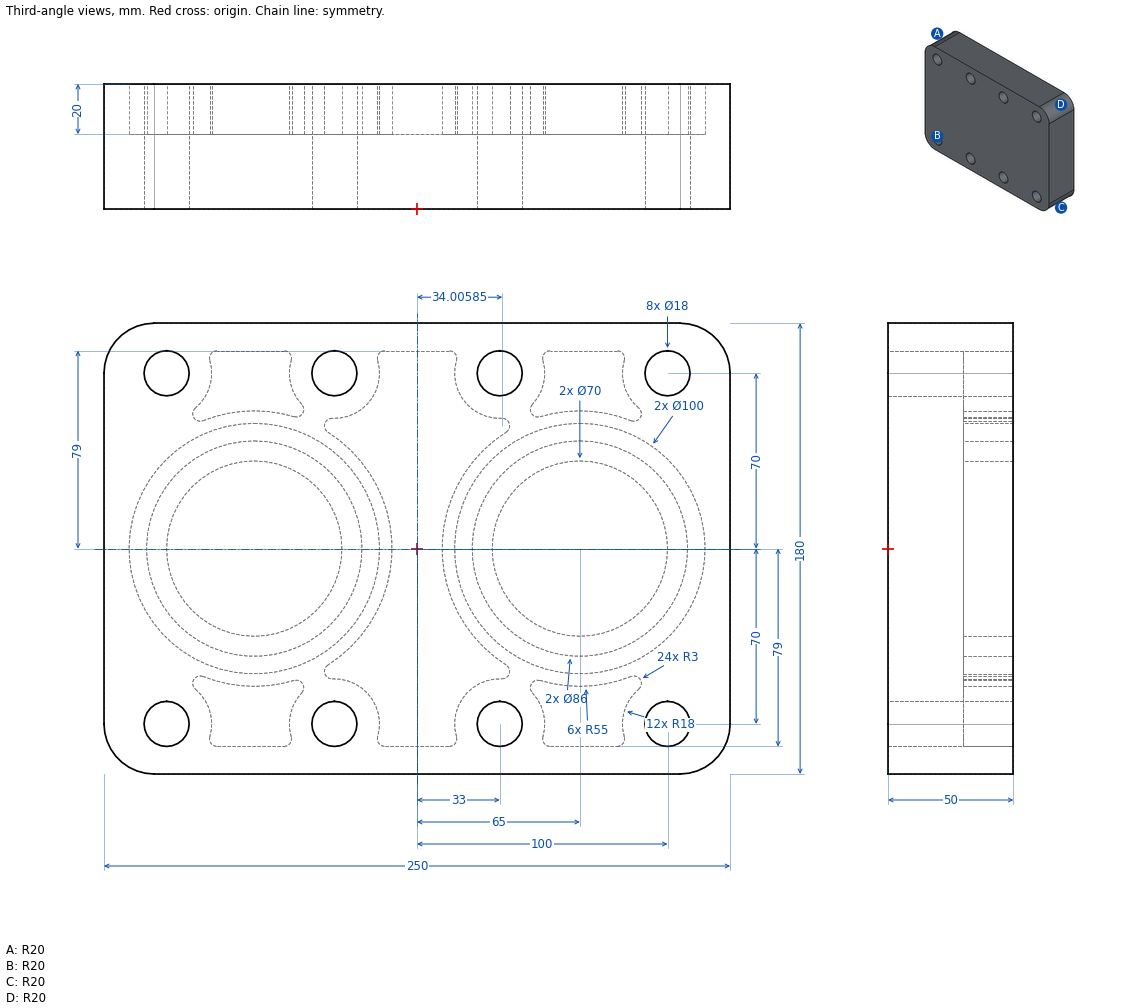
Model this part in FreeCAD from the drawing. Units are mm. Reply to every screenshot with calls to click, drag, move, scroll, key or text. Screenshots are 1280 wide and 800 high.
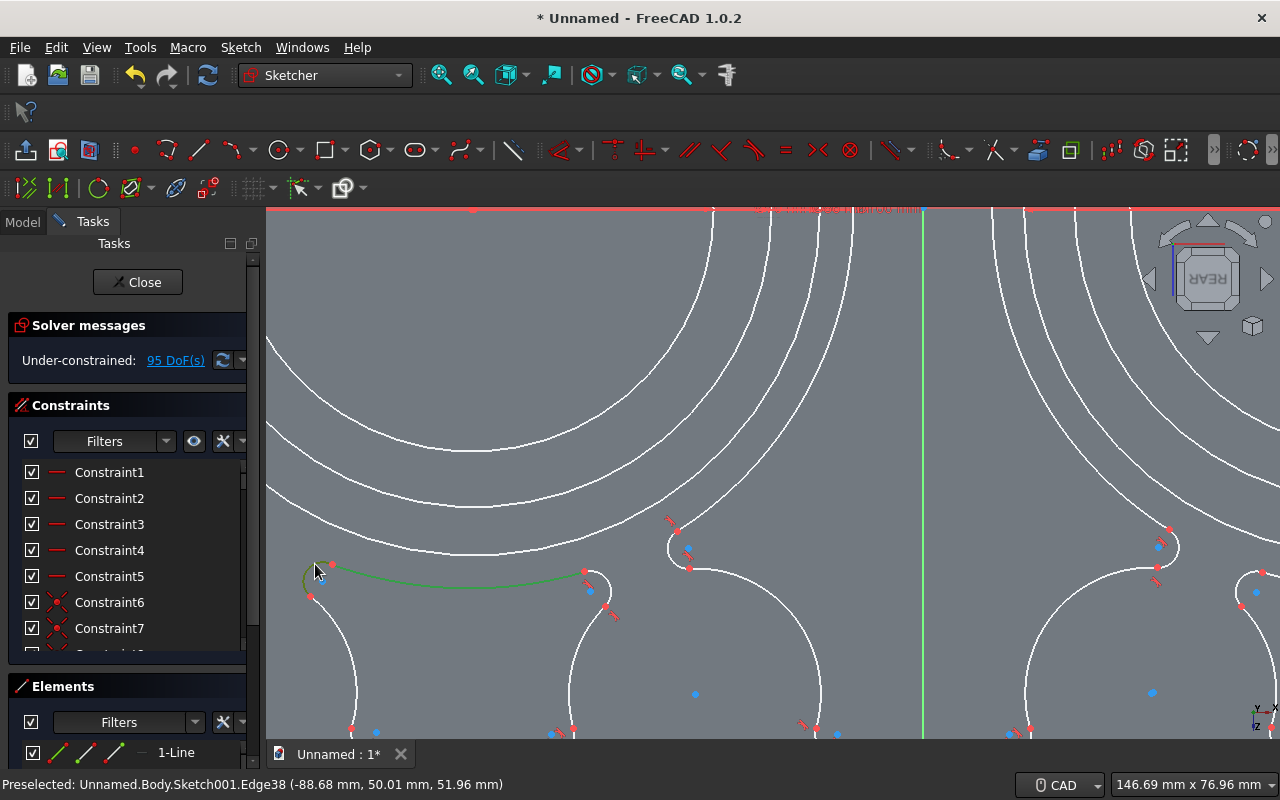
click(754, 150)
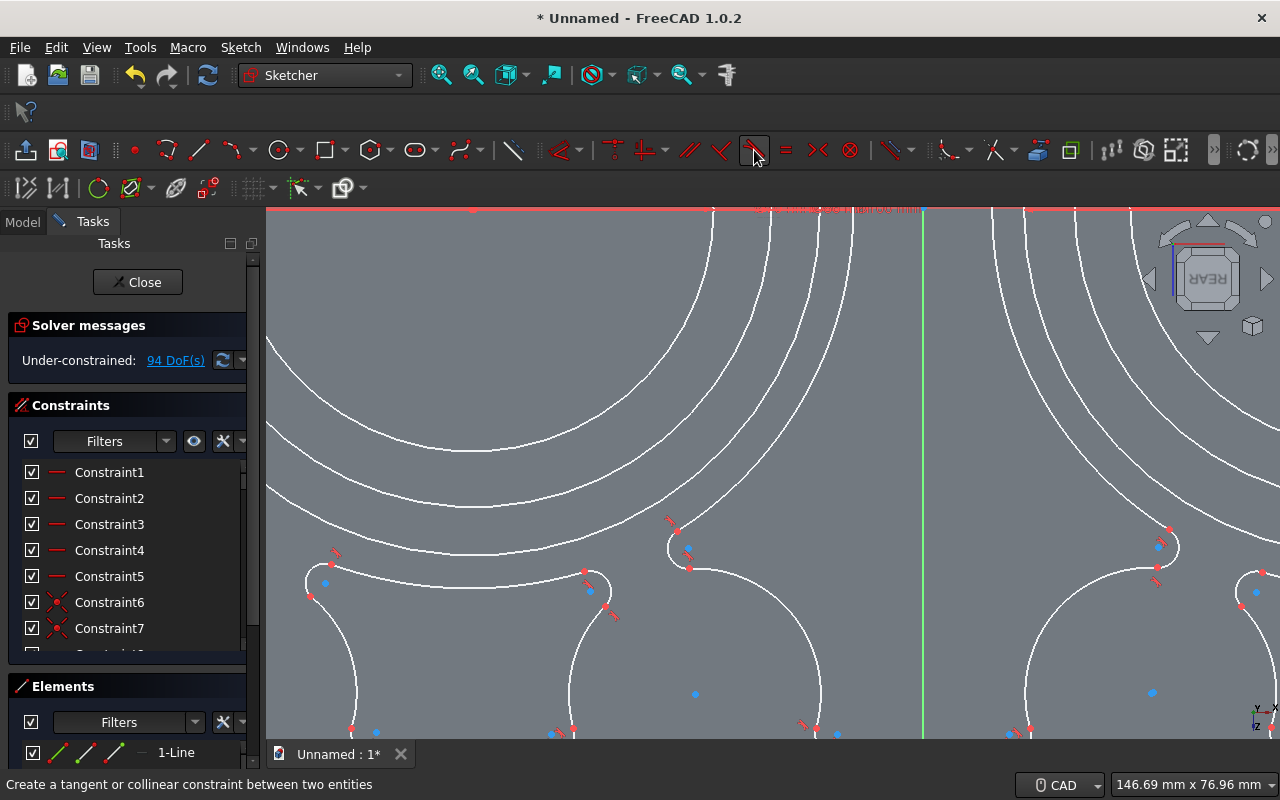
click(317, 566)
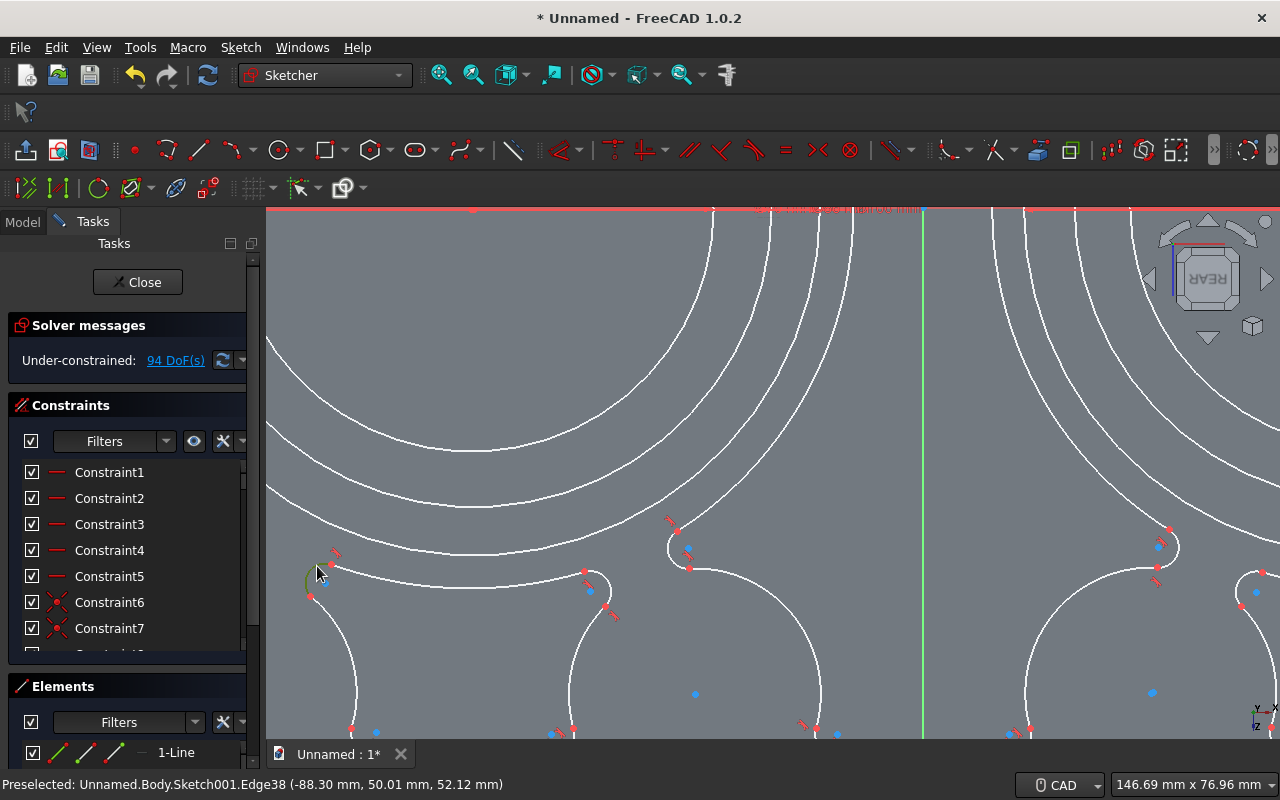
scroll(610, 587, down, 6)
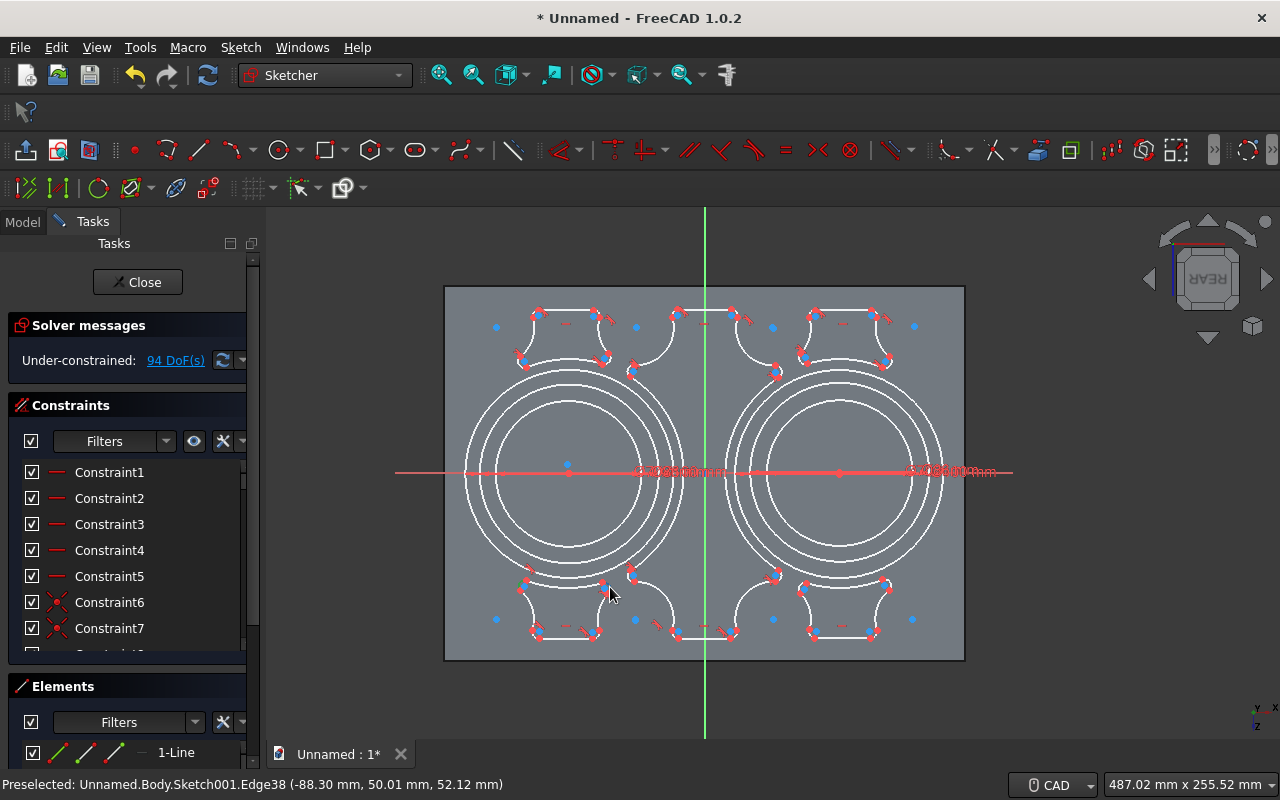
click(534, 617)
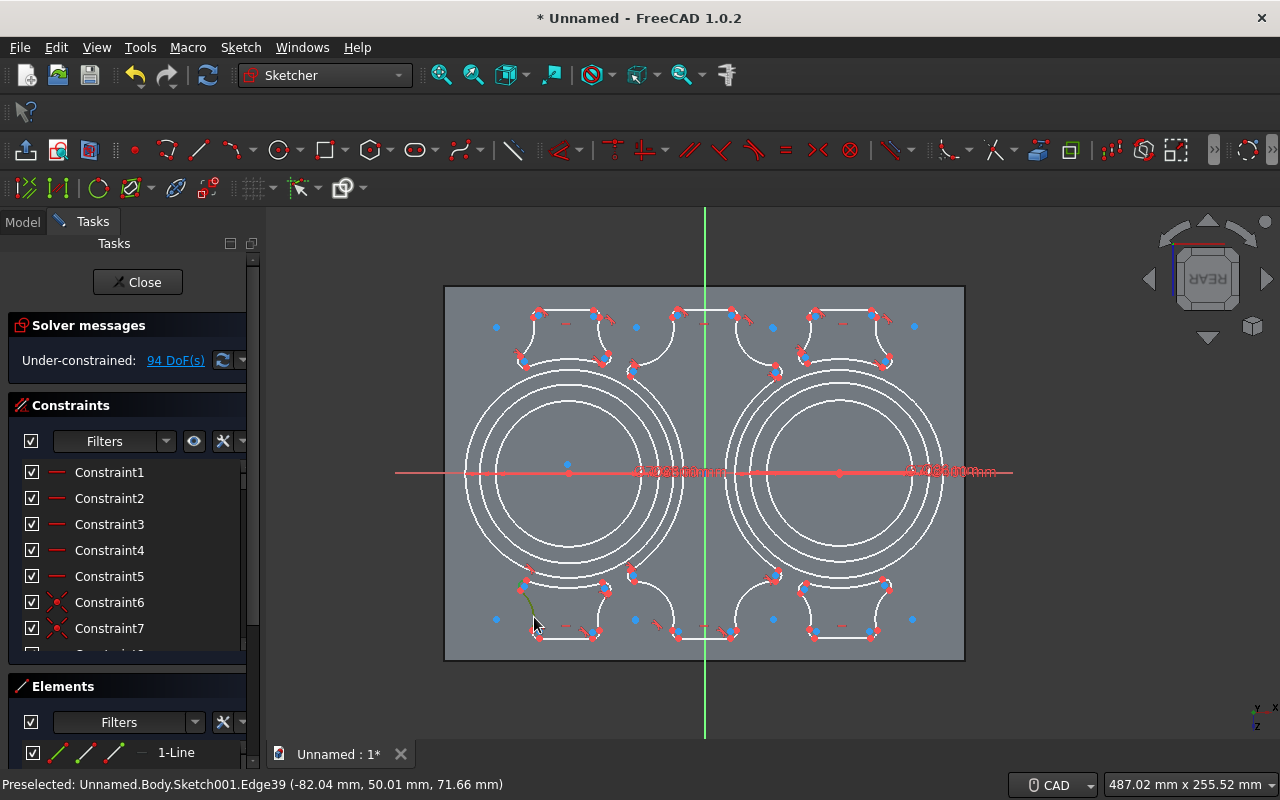
click(754, 150)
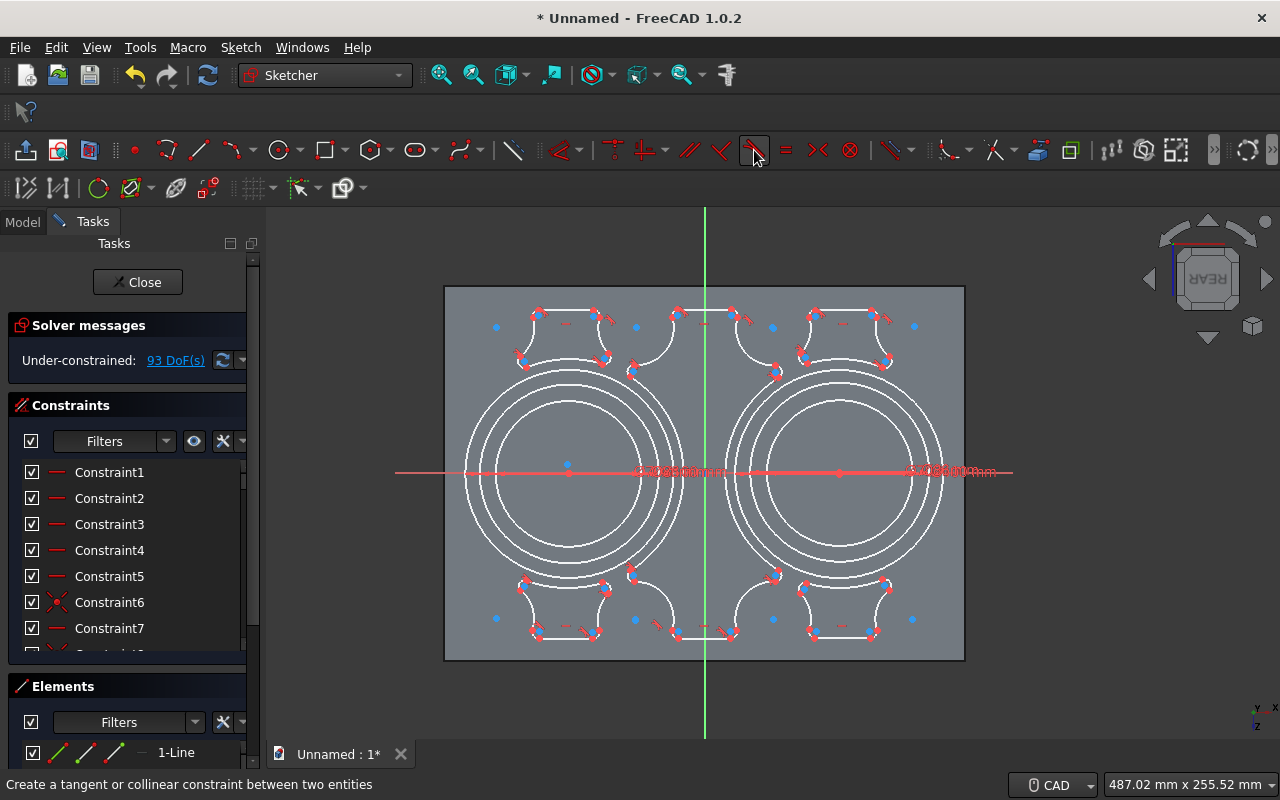
click(534, 617)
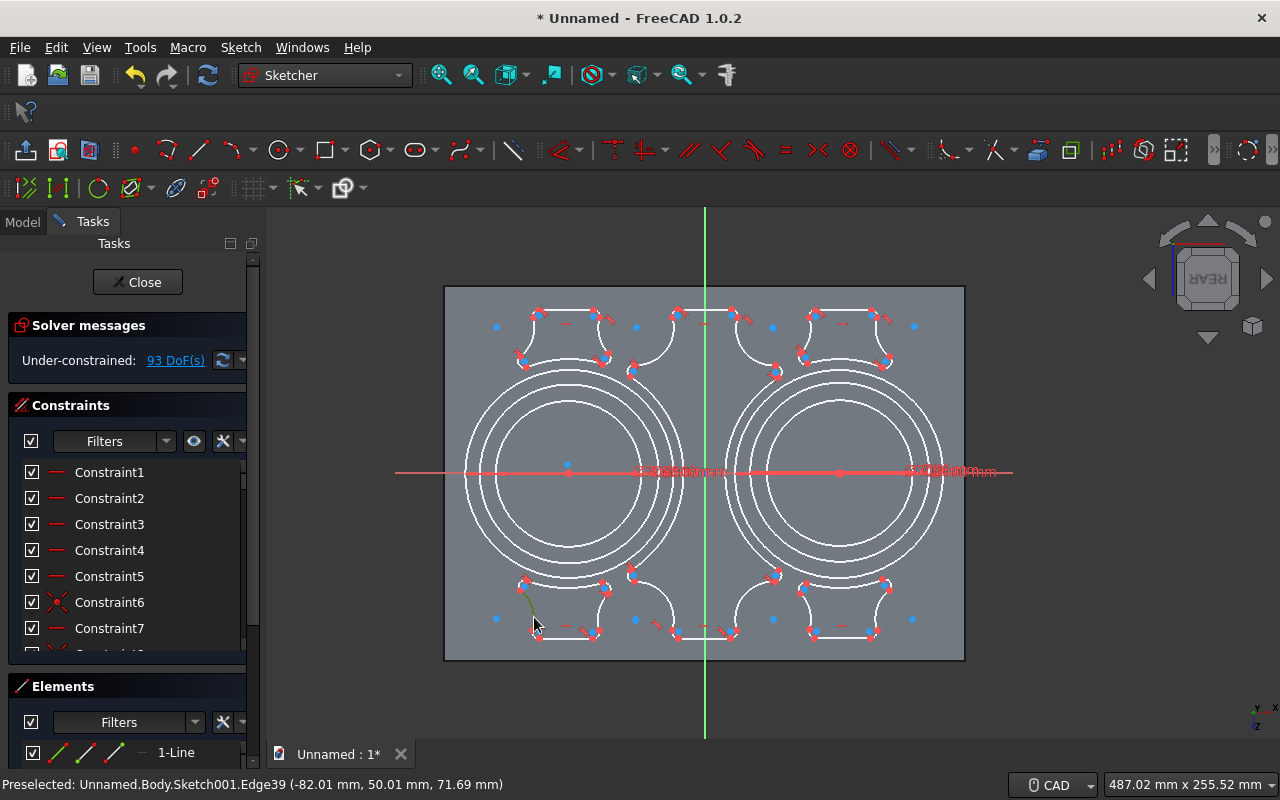
scroll(534, 636, up, 4)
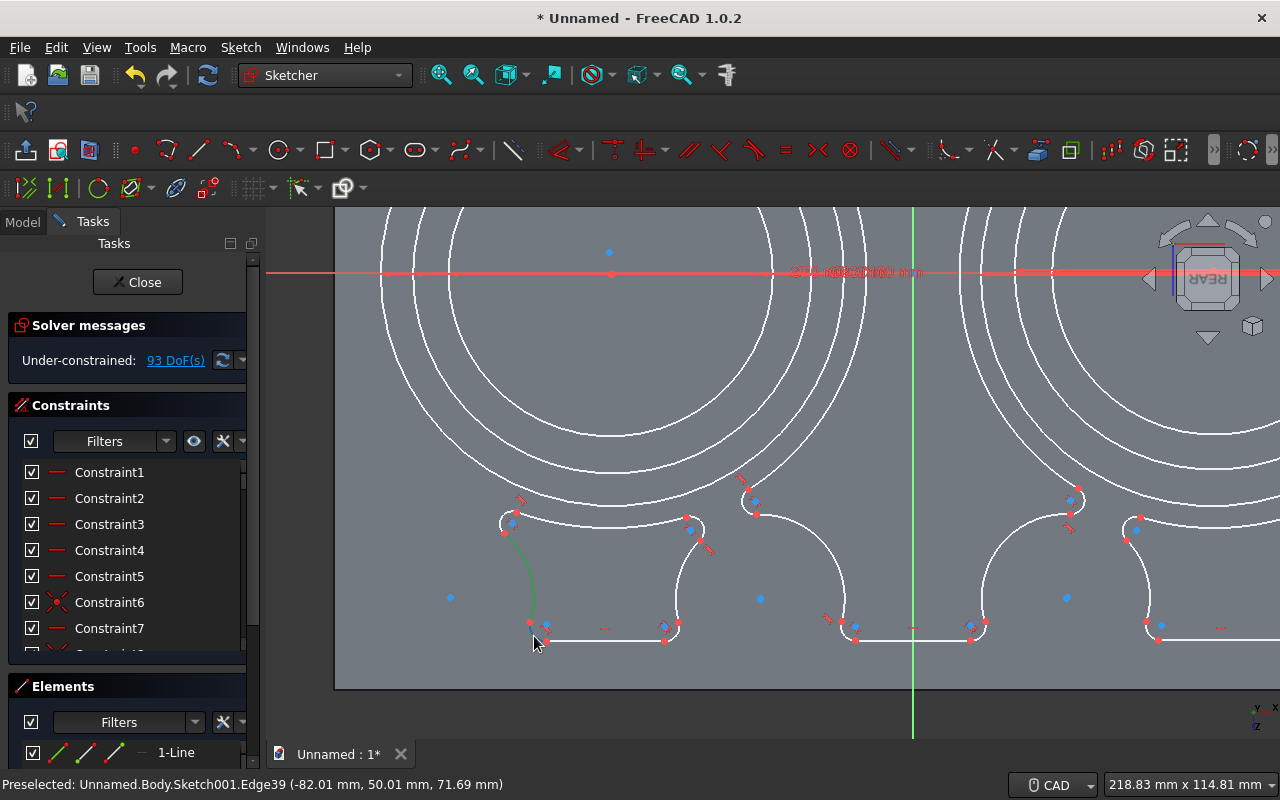
click(534, 636)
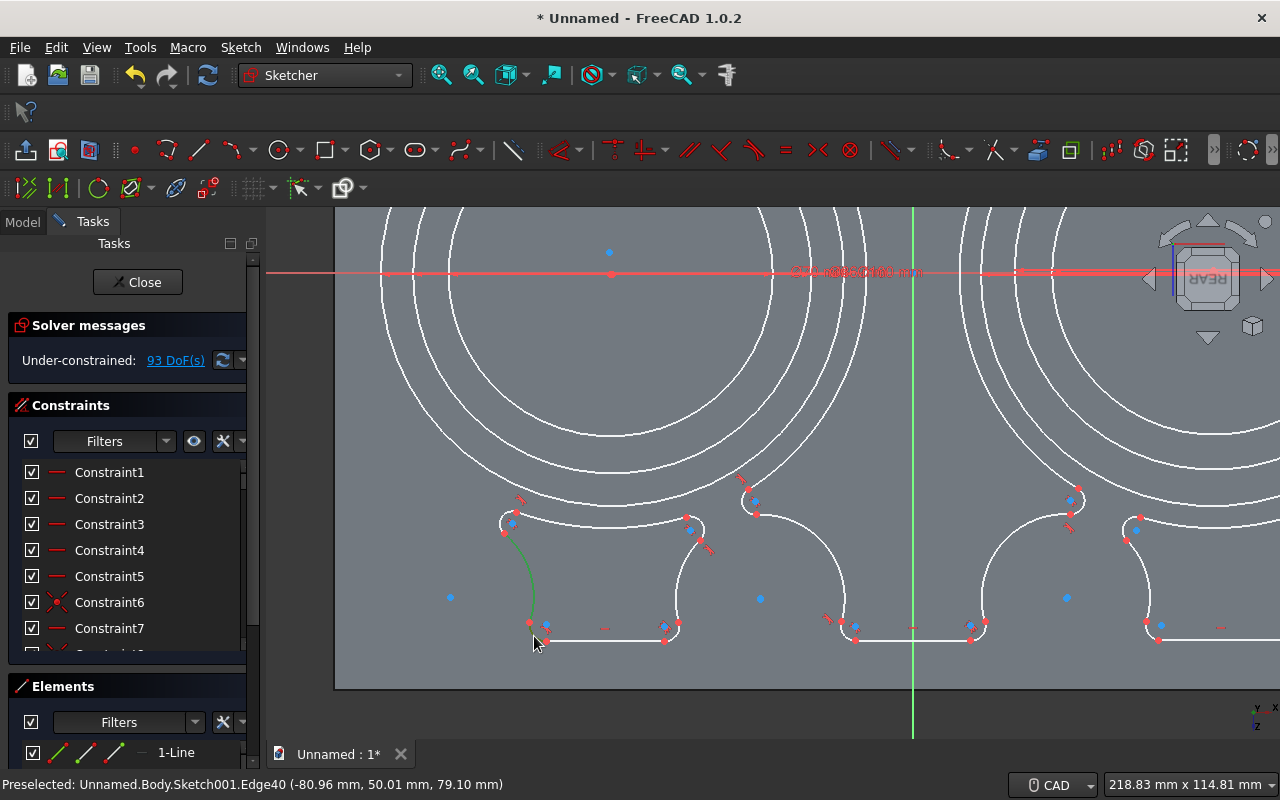
click(754, 150)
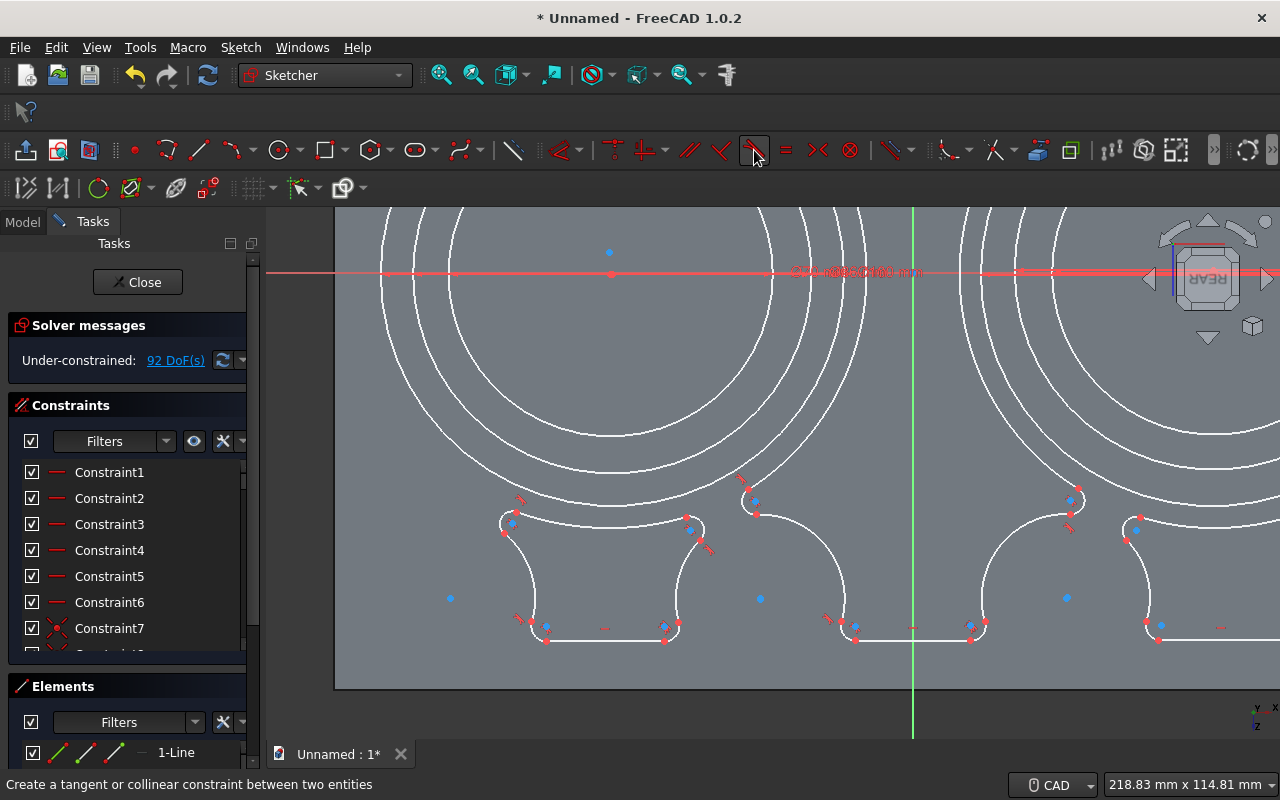
scroll(534, 636, down, 4)